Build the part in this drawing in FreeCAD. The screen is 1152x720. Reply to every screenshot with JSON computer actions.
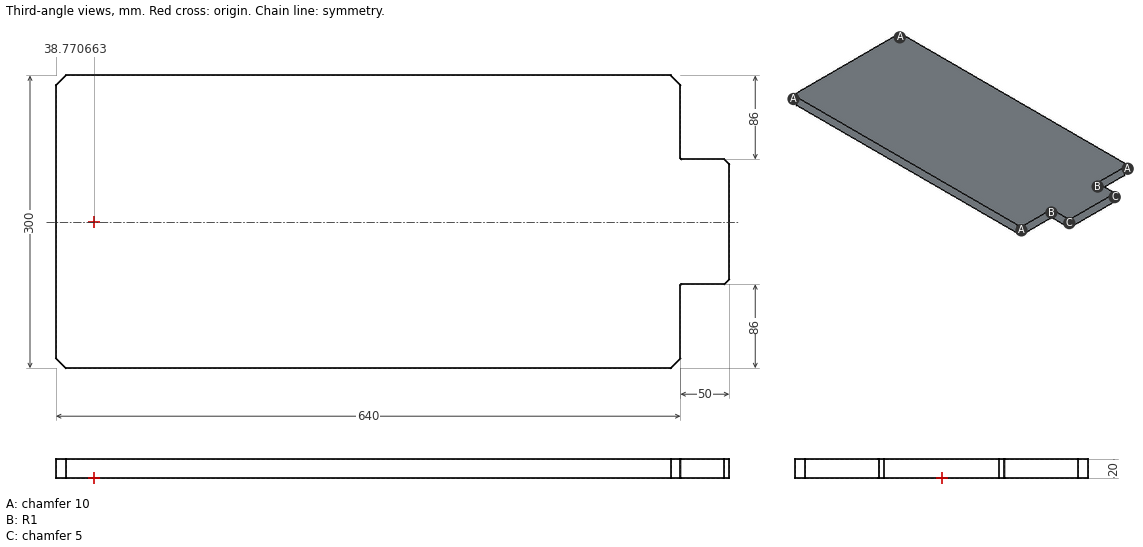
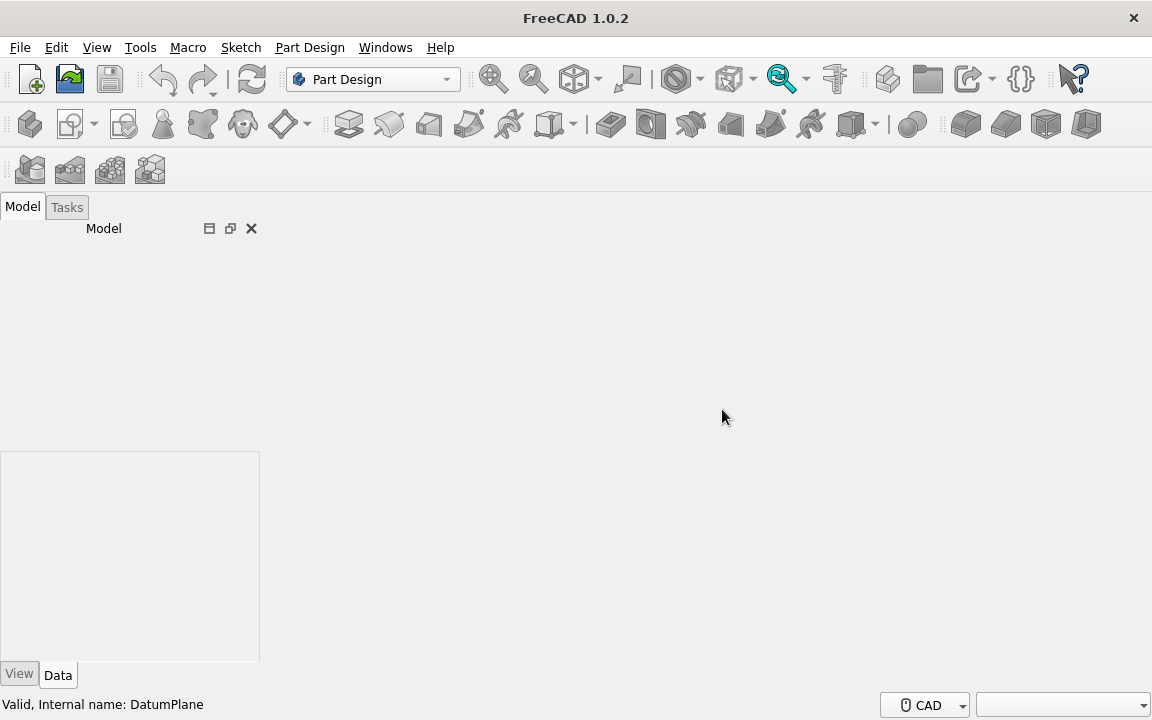
{"action": "left_click", "coordinate": [30, 80]}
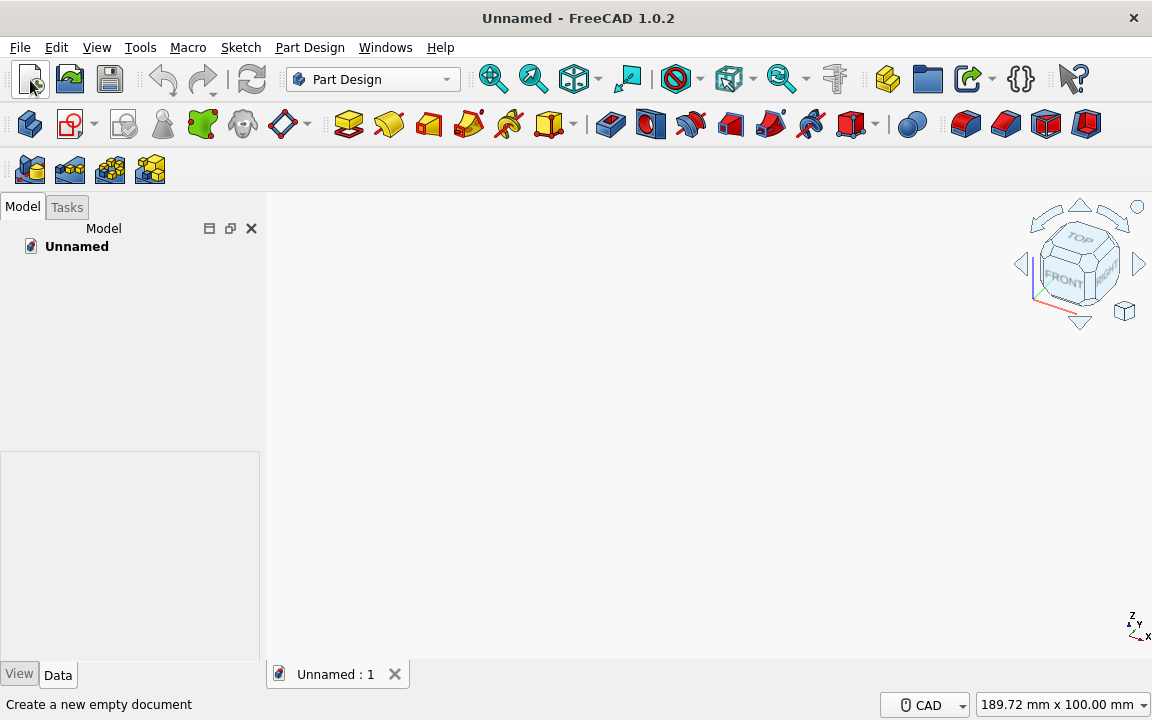
{"action": "left_click", "coordinate": [70, 124]}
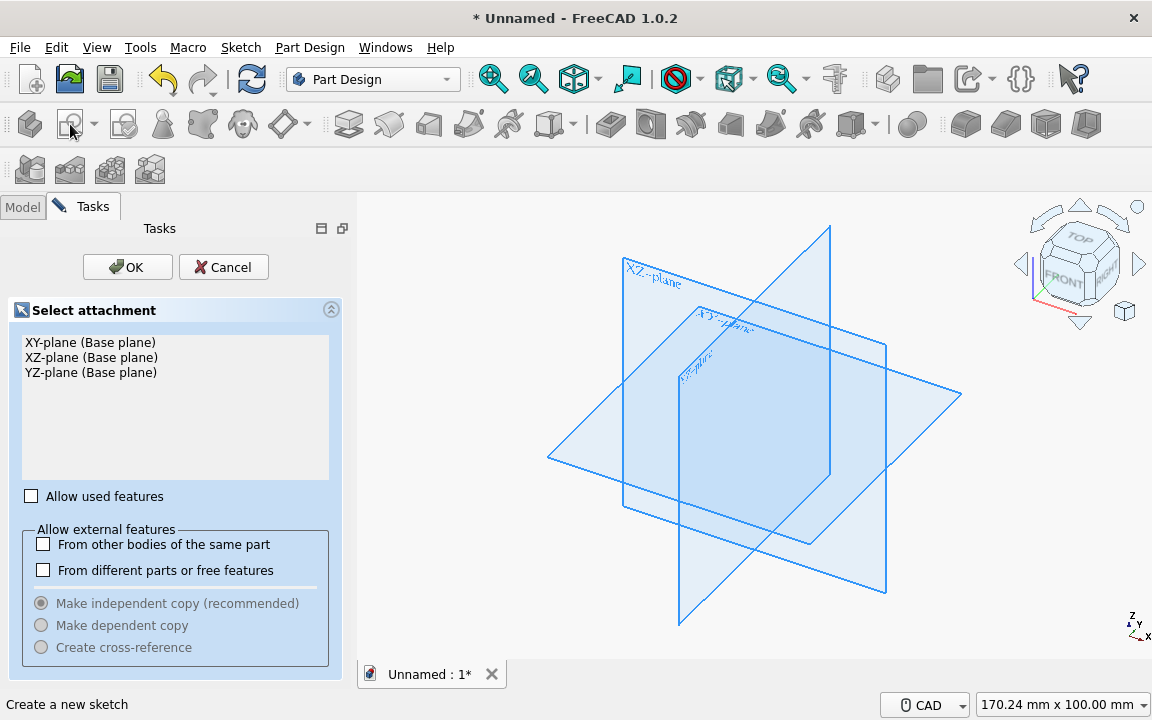
{"action": "left_click", "coordinate": [82, 342]}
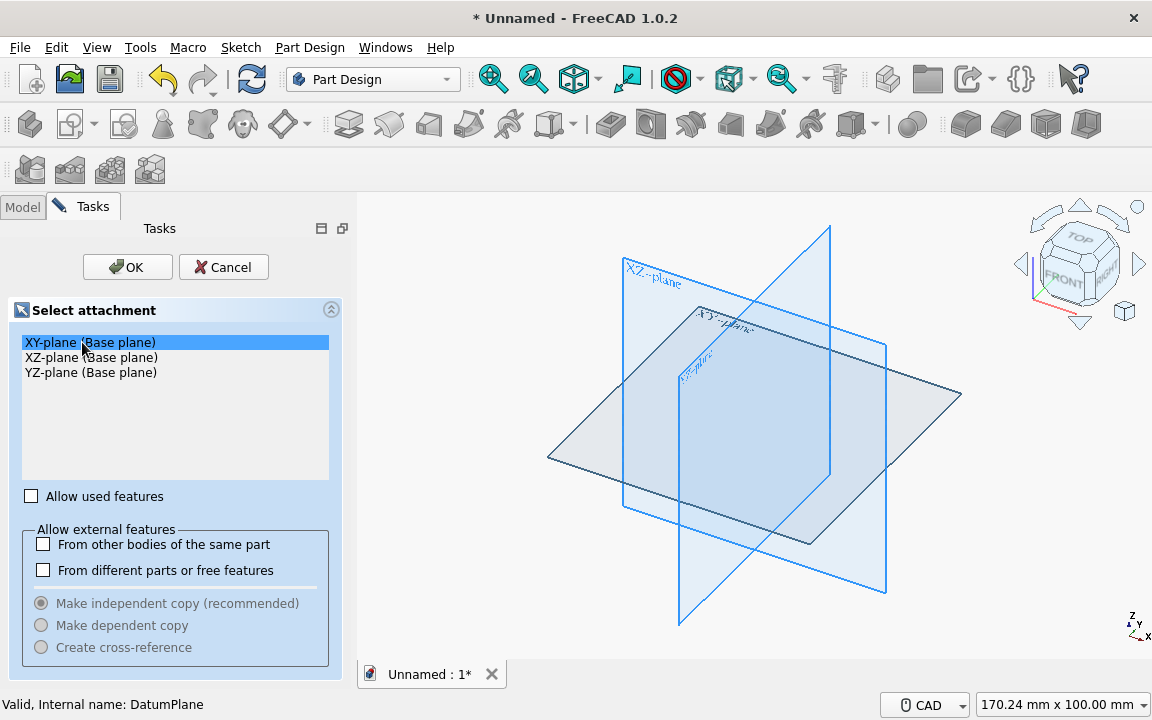
{"action": "left_click", "coordinate": [128, 267]}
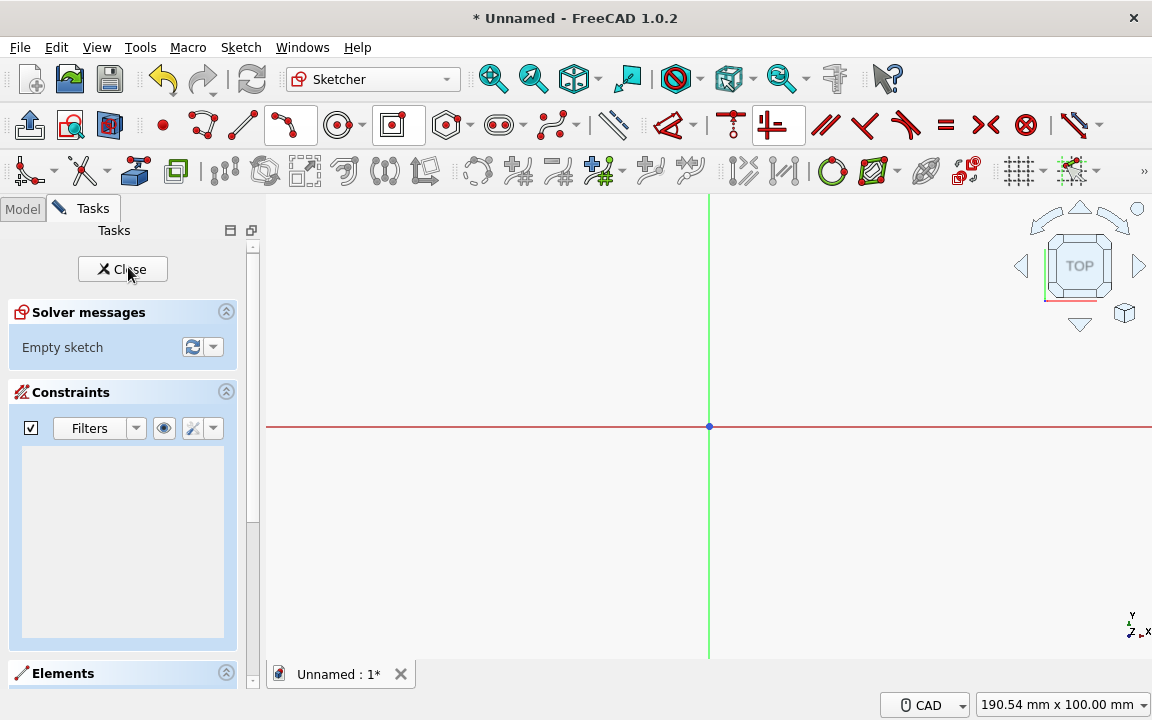
{"action": "scroll", "coordinate": [345, 426], "scroll_direction": "down", "scroll_amount": 9}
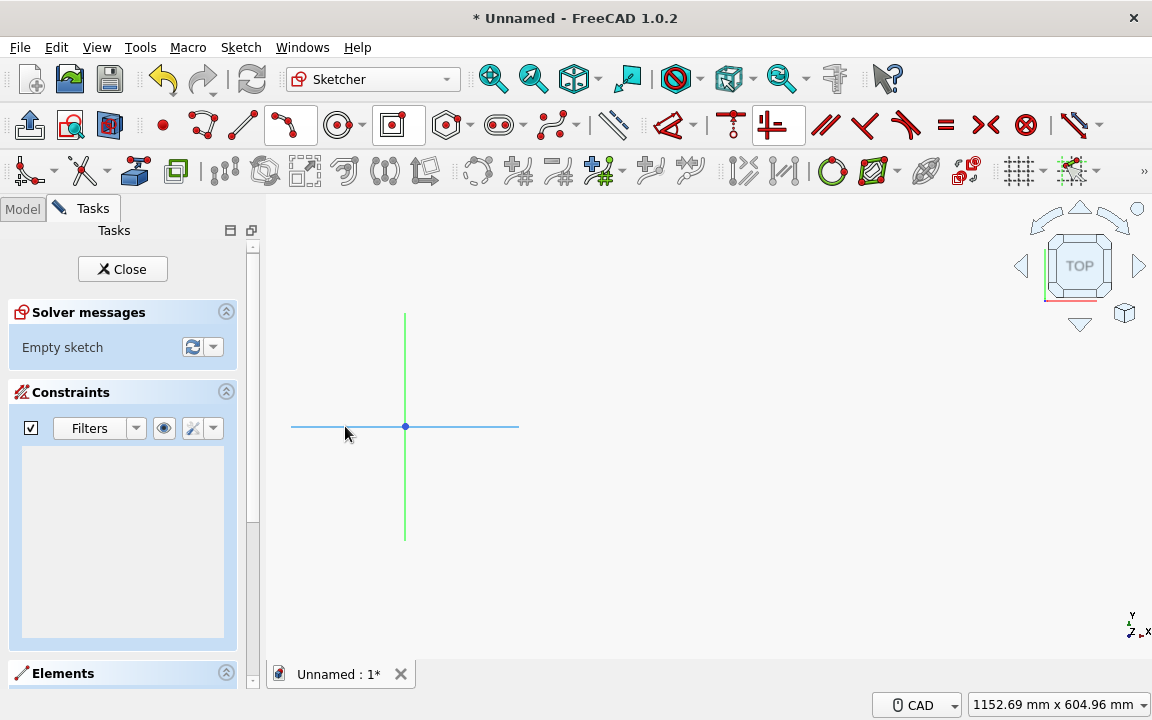
{"action": "key", "text": "g m"}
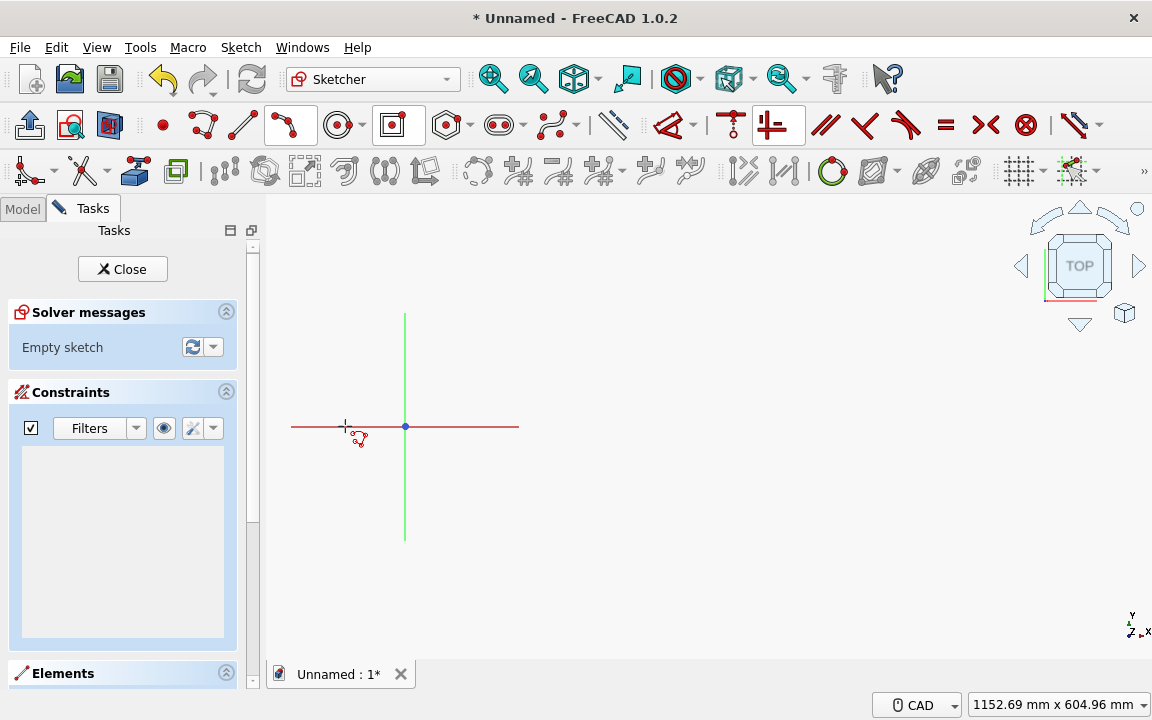
{"action": "left_click", "coordinate": [375, 311]}
{"action": "left_click", "coordinate": [375, 542]}
{"action": "left_click", "coordinate": [867, 542]}
{"action": "left_click", "coordinate": [867, 476]}
{"action": "left_click", "coordinate": [906, 476]}
{"action": "left_click", "coordinate": [906, 377]}
{"action": "left_click", "coordinate": [867, 377]}
{"action": "left_click", "coordinate": [867, 311]}
{"action": "left_click", "coordinate": [375, 312]}
{"action": "key", "text": "Escape"}
{"action": "key", "text": "Escape"}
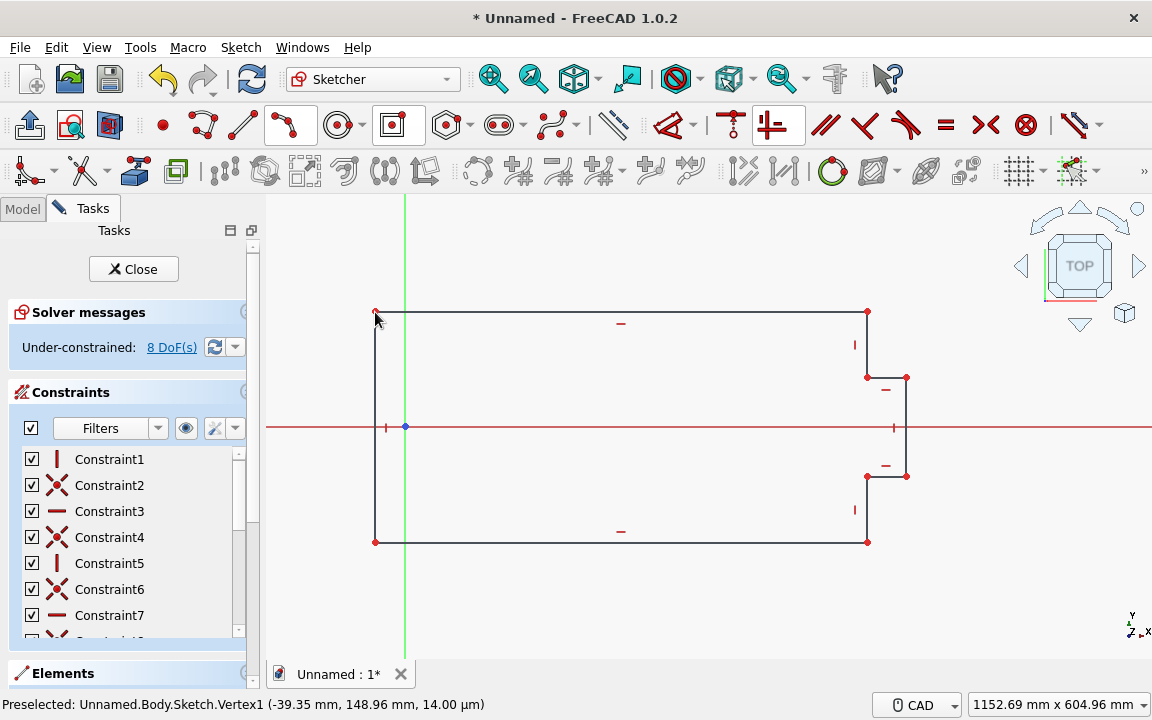
{"action": "left_click", "coordinate": [867, 477]}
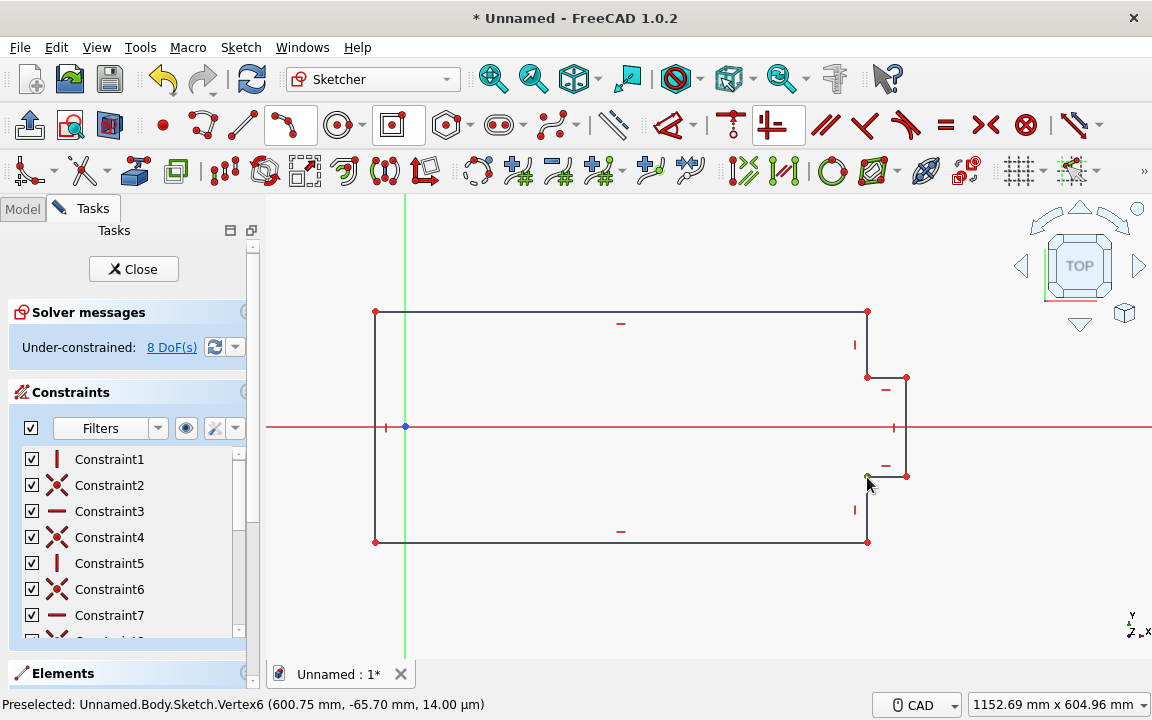
{"action": "left_click", "coordinate": [867, 378]}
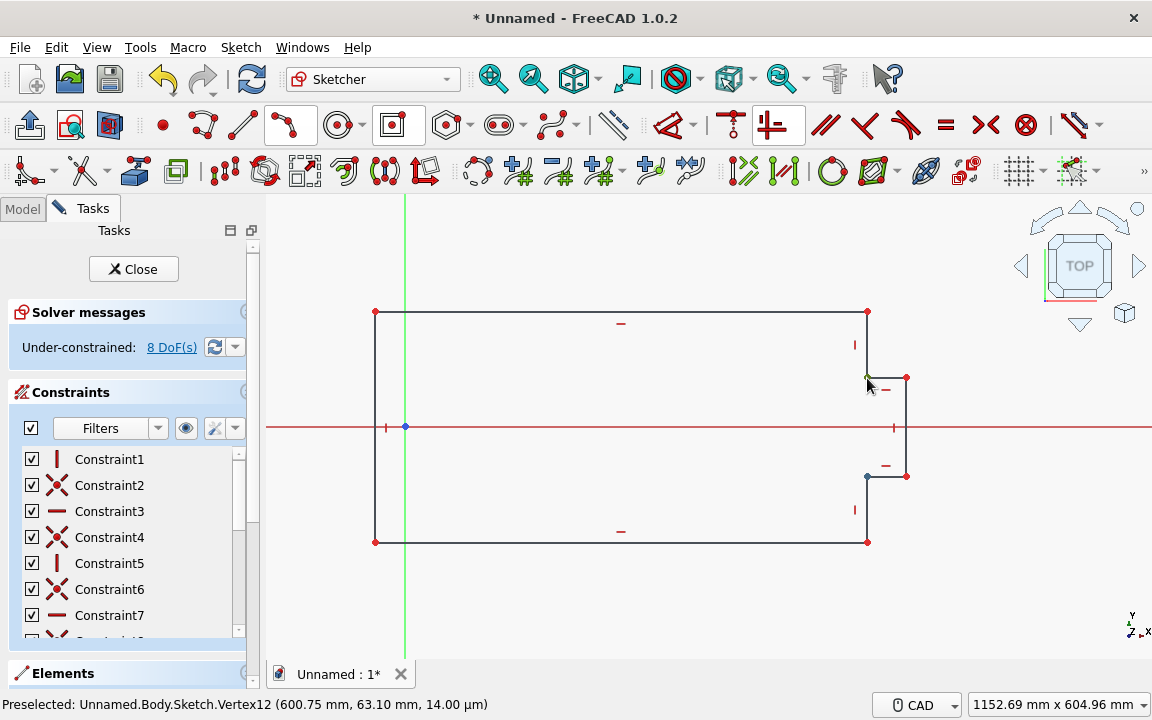
{"action": "left_click", "coordinate": [344, 426]}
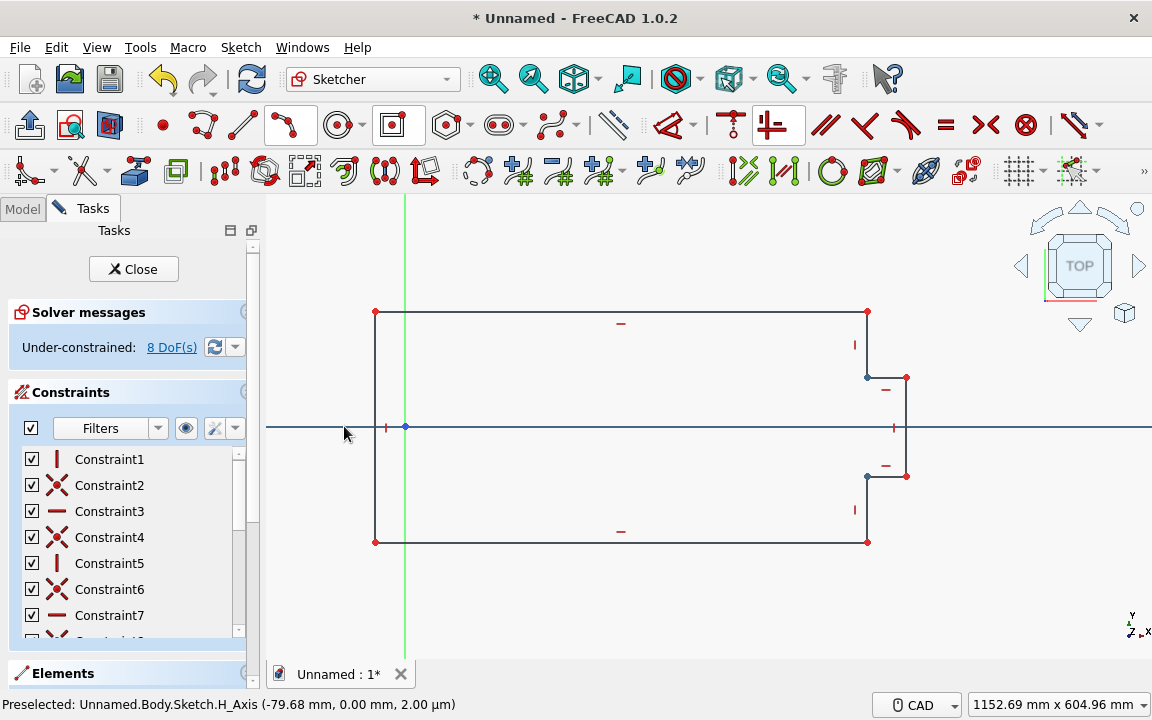
{"action": "left_click", "coordinate": [986, 126]}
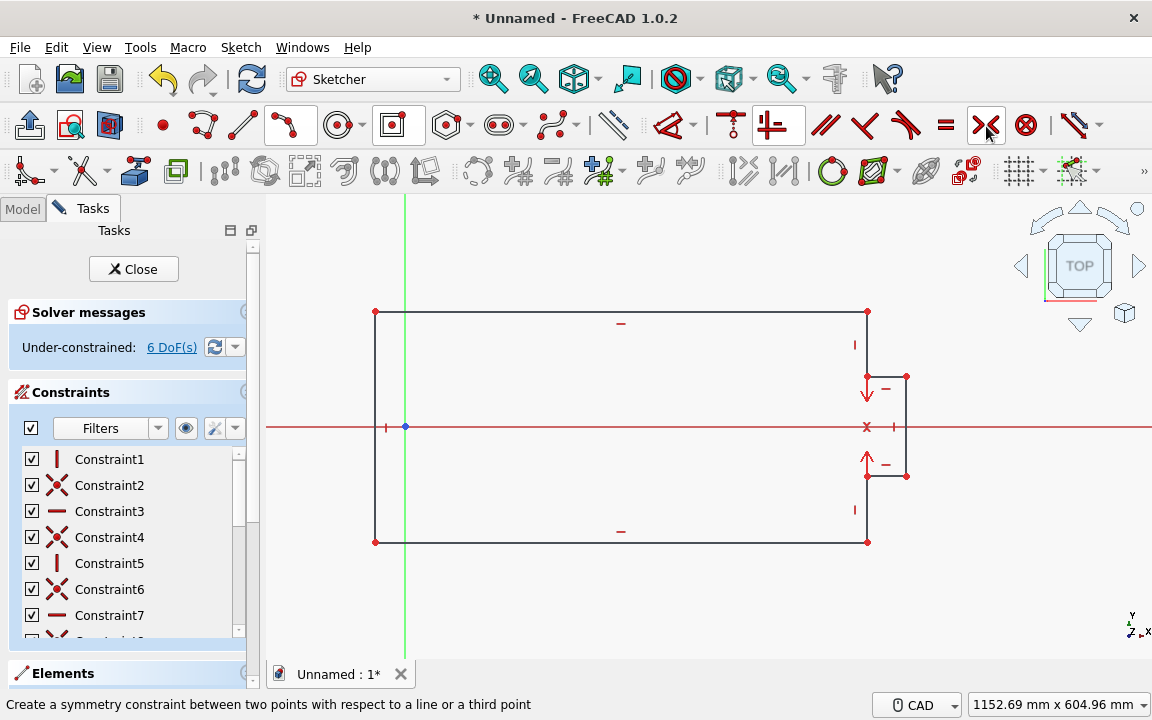
{"action": "left_click", "coordinate": [668, 126]}